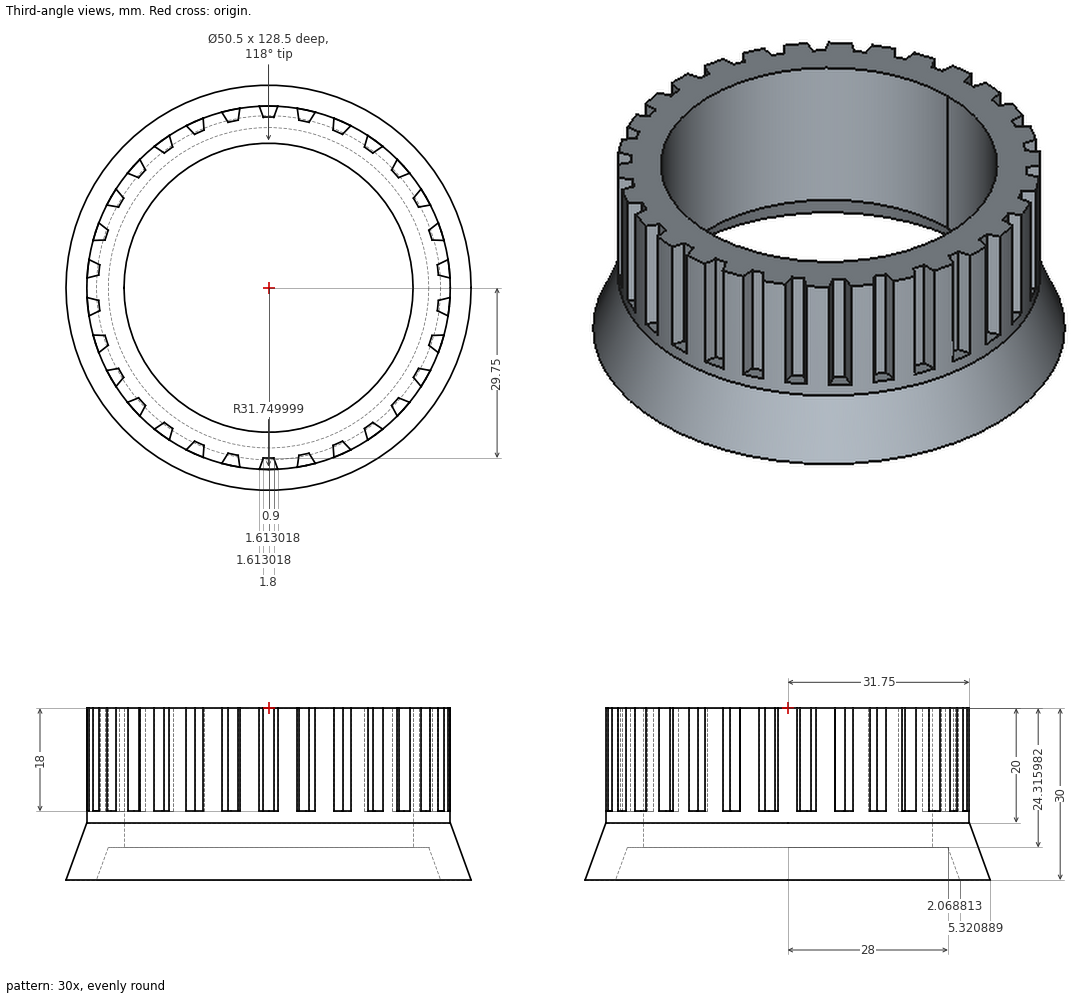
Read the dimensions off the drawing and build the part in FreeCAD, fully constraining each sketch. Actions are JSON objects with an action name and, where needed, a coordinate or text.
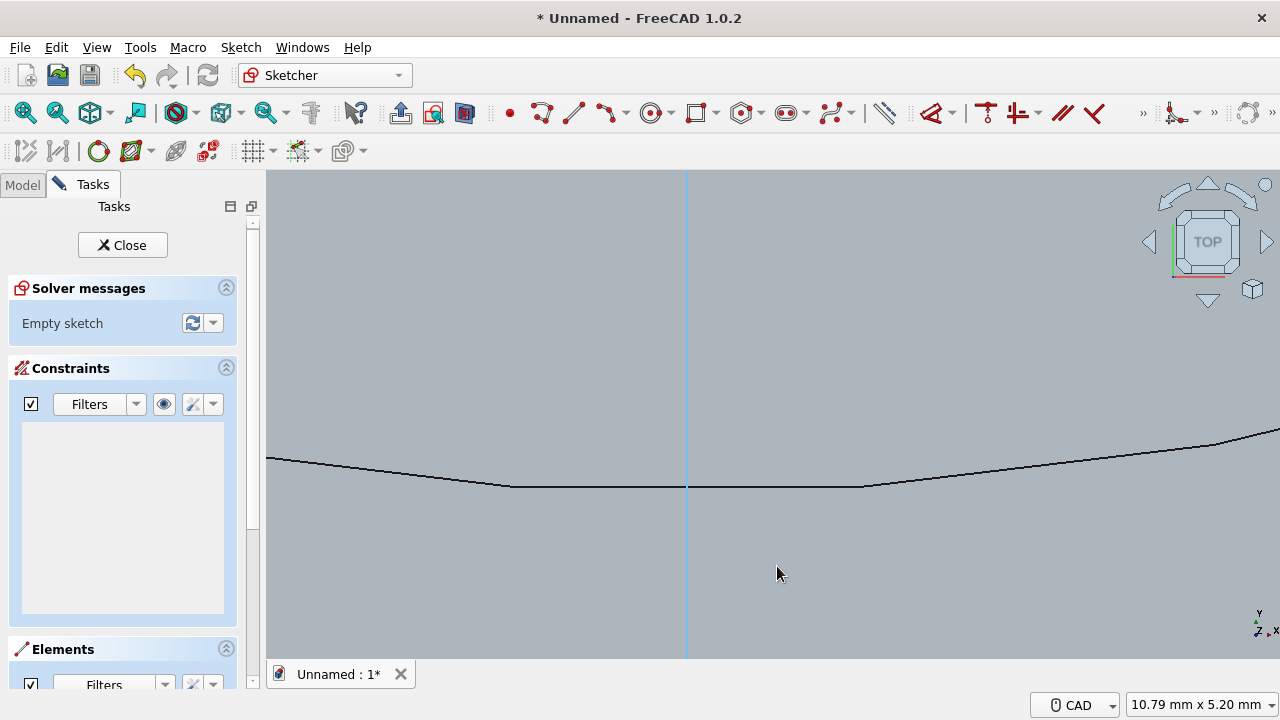
{"action": "scroll", "coordinate": [652, 364], "scroll_direction": "up", "scroll_amount": 2}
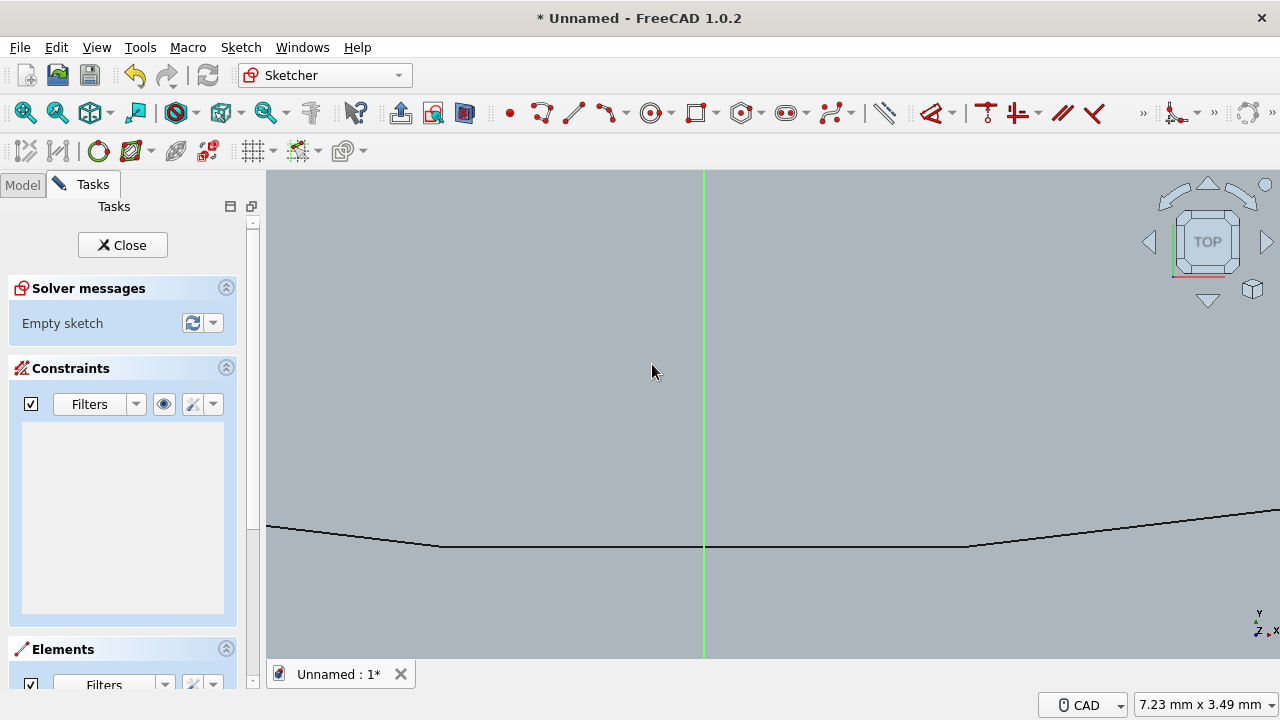
{"action": "left_click", "coordinate": [542, 114]}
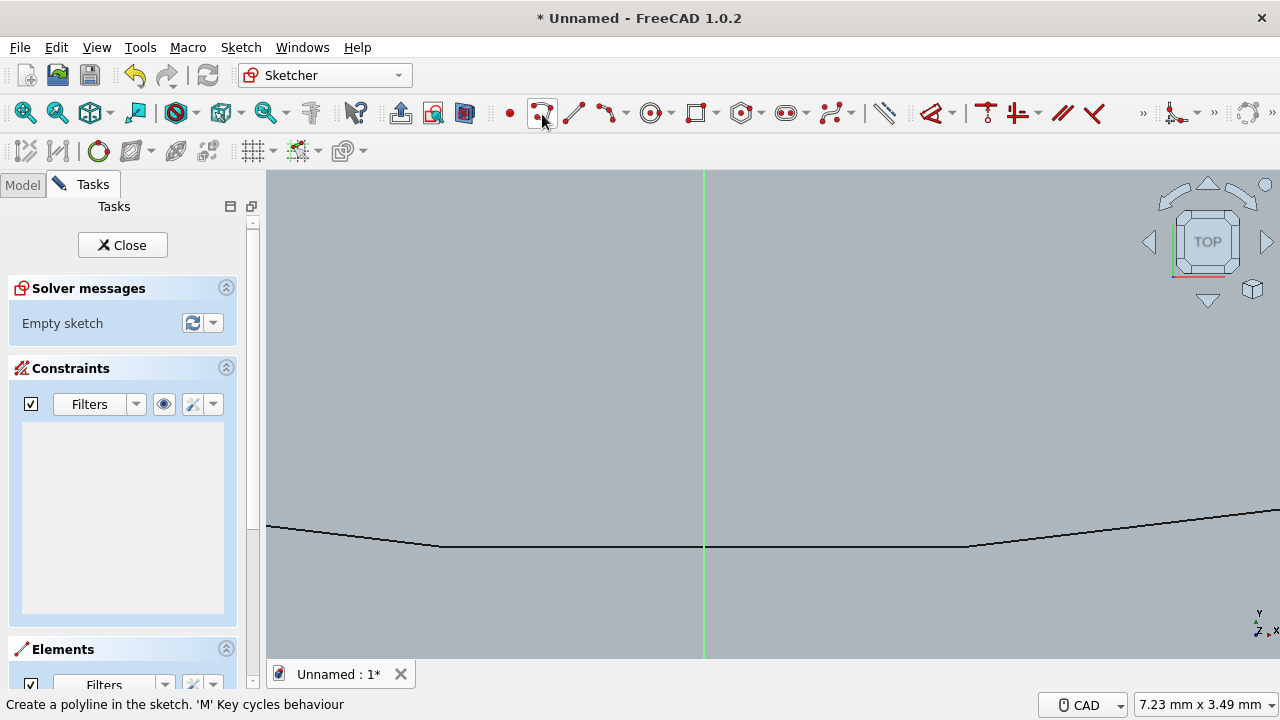
{"action": "left_click", "coordinate": [930, 549]}
{"action": "left_click", "coordinate": [830, 274]}
{"action": "left_click", "coordinate": [578, 274]}
{"action": "left_click", "coordinate": [478, 549]}
{"action": "right_click", "coordinate": [478, 549]}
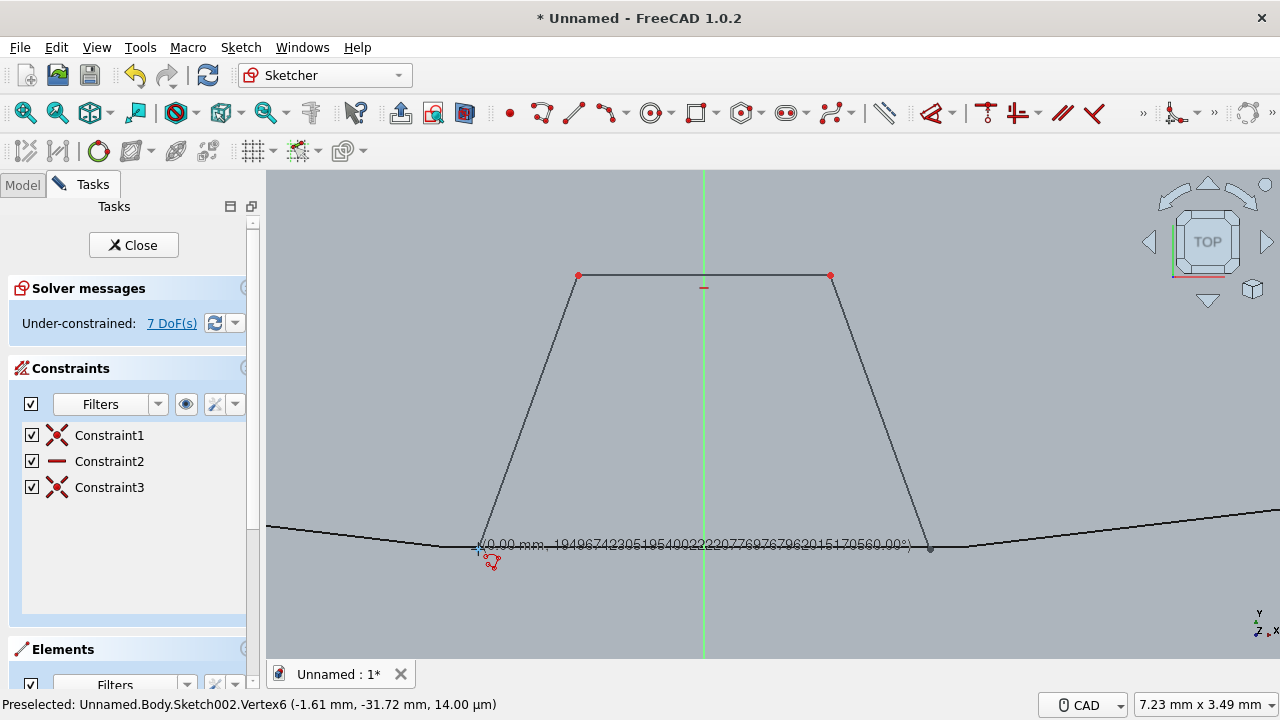
{"action": "left_click", "coordinate": [606, 114]}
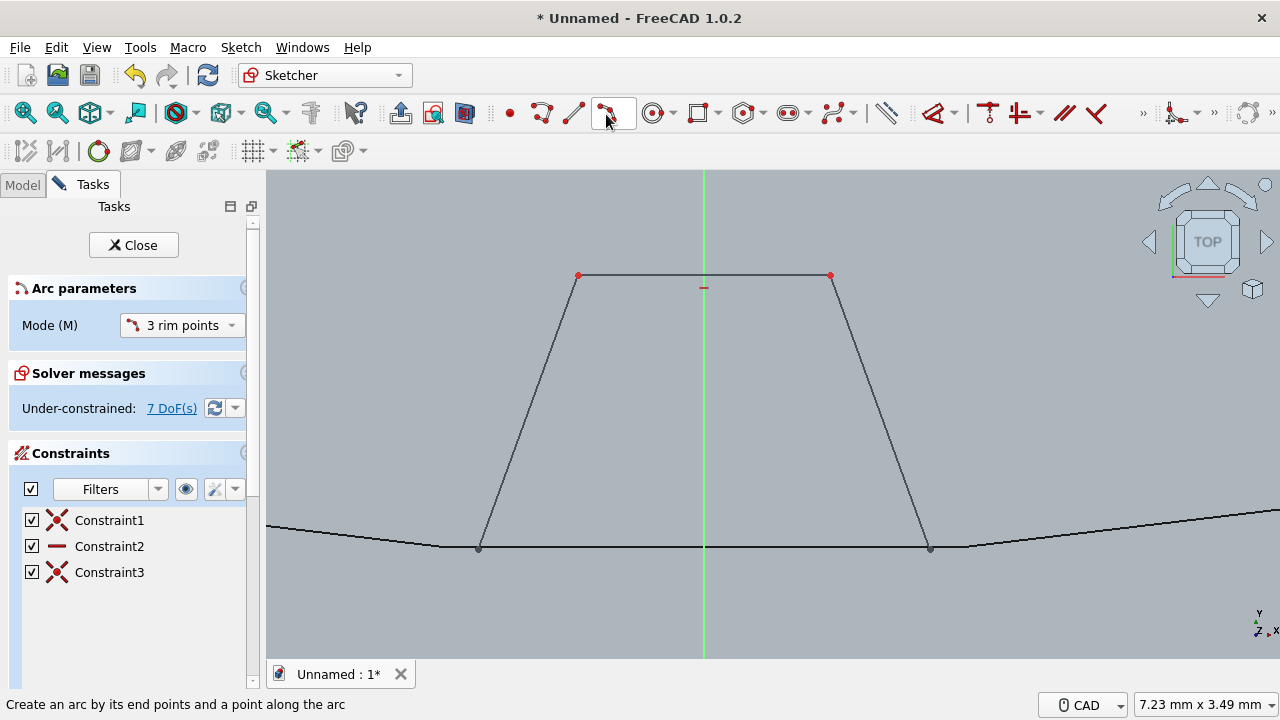
{"action": "left_click", "coordinate": [478, 550]}
{"action": "left_click", "coordinate": [930, 550]}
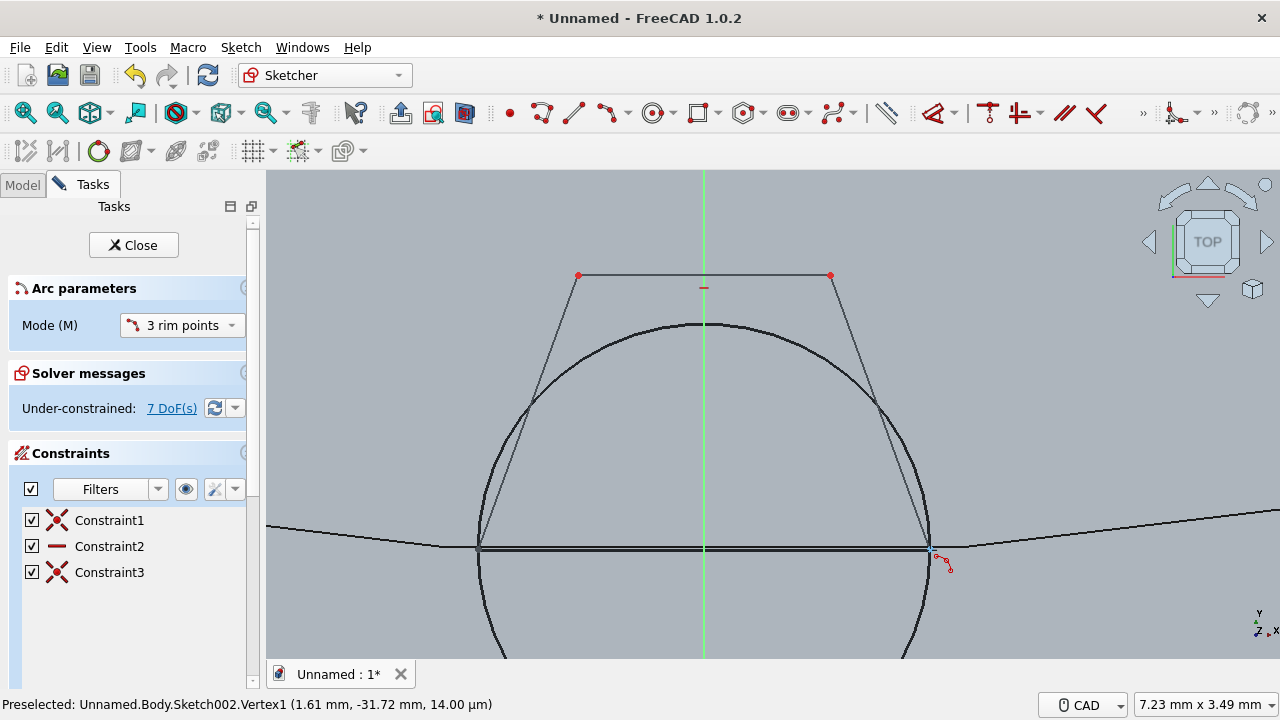
{"action": "scroll", "coordinate": [659, 554], "scroll_direction": "up", "scroll_amount": 6}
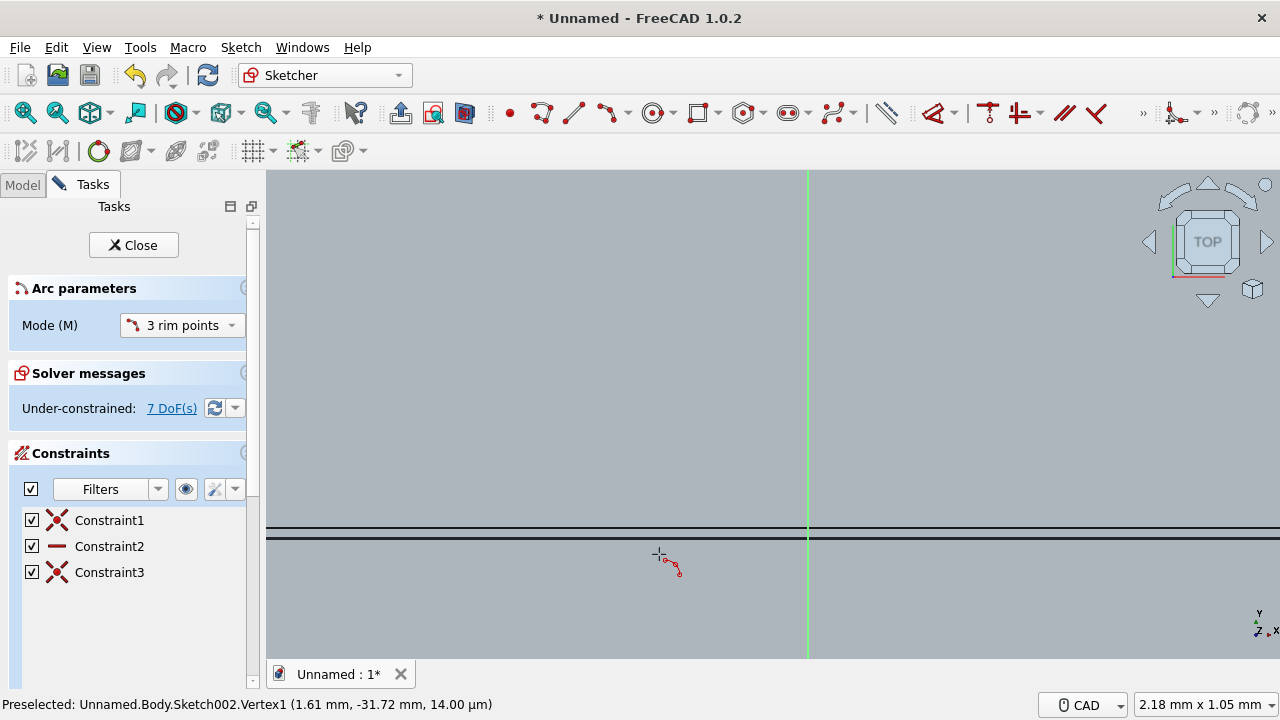
{"action": "left_click", "coordinate": [657, 553]}
{"action": "key", "text": "Escape"}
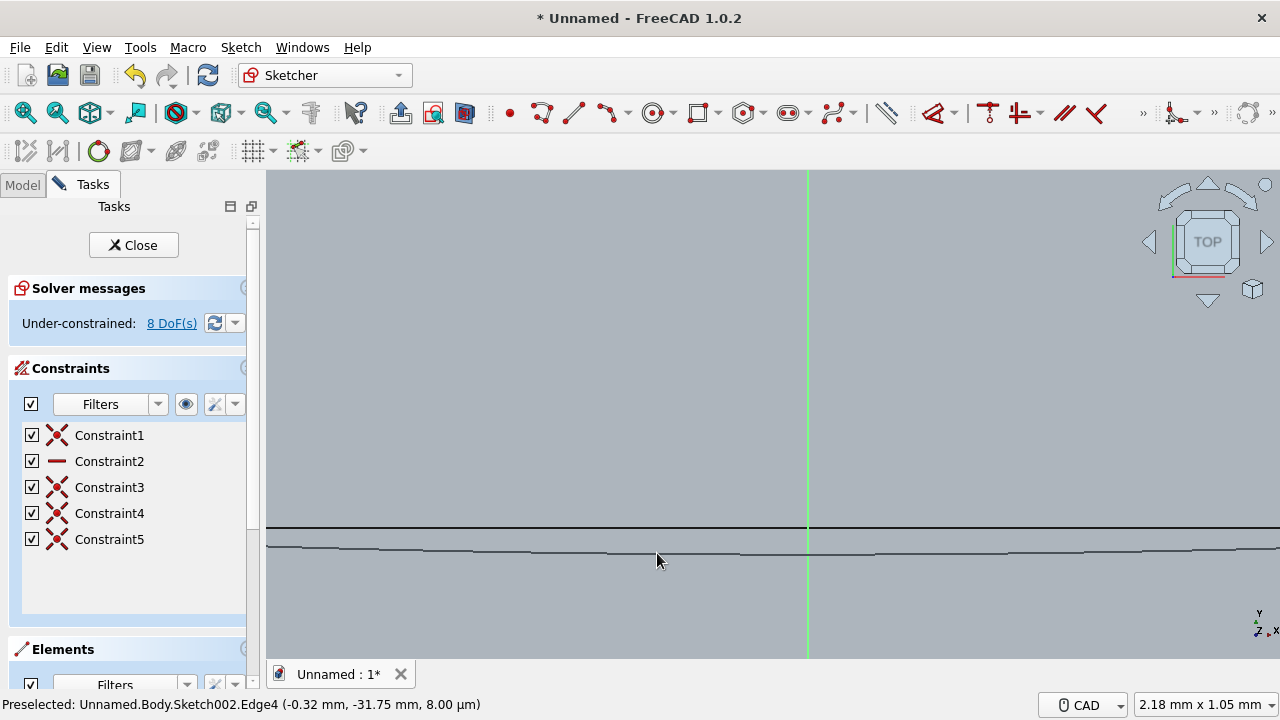
{"action": "scroll", "coordinate": [660, 555], "scroll_direction": "down", "scroll_amount": 6}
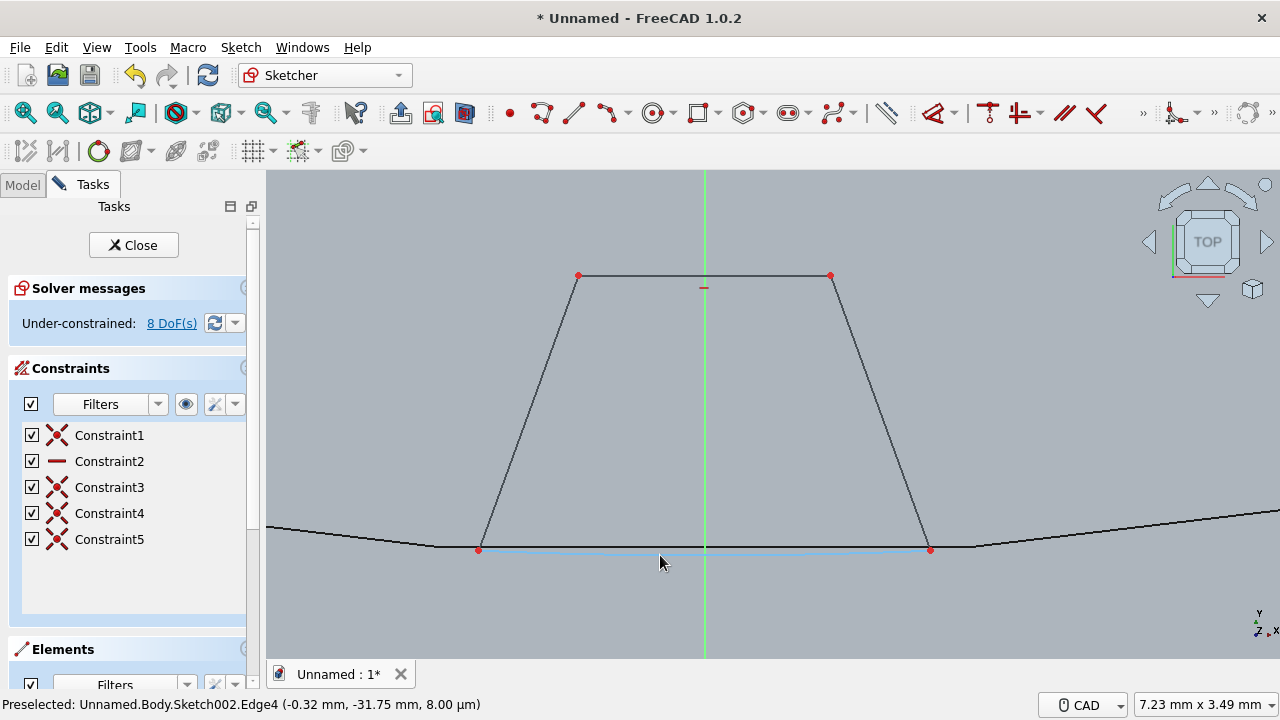
{"action": "scroll", "coordinate": [704, 565], "scroll_direction": "down", "scroll_amount": 14}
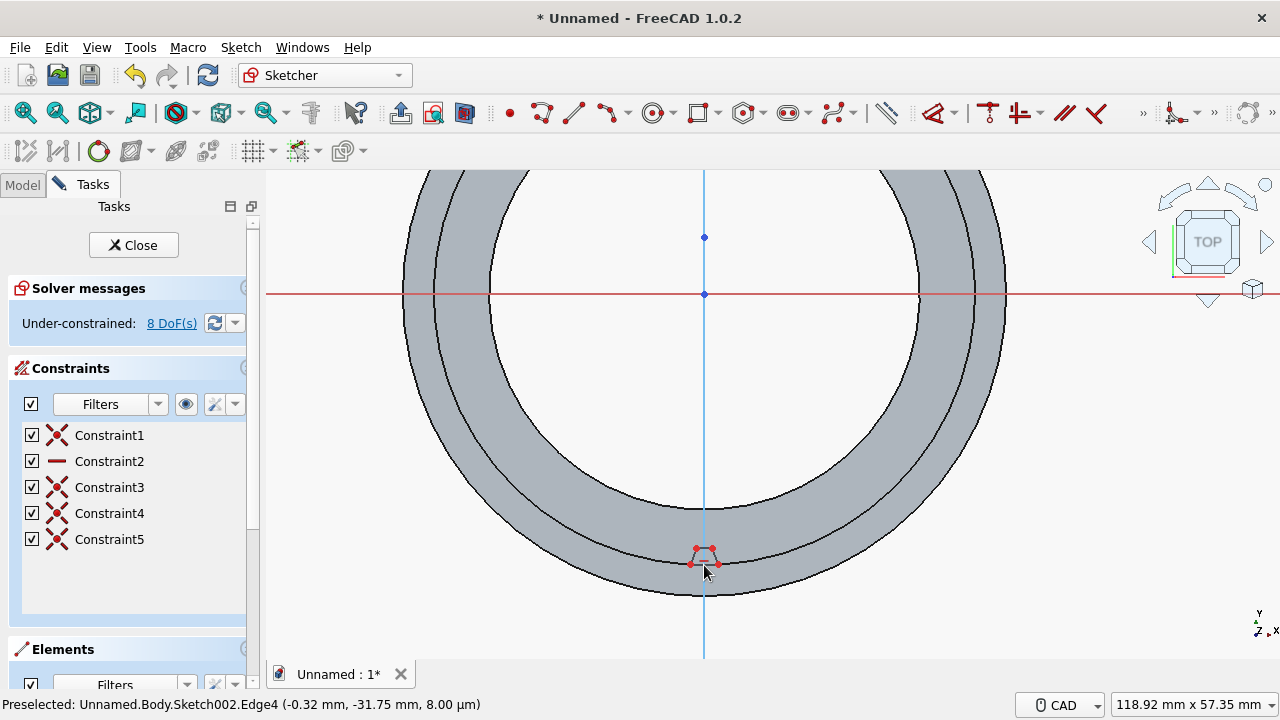
{"action": "left_click_drag", "start_coordinate": [694, 228], "coordinate": [714, 304]}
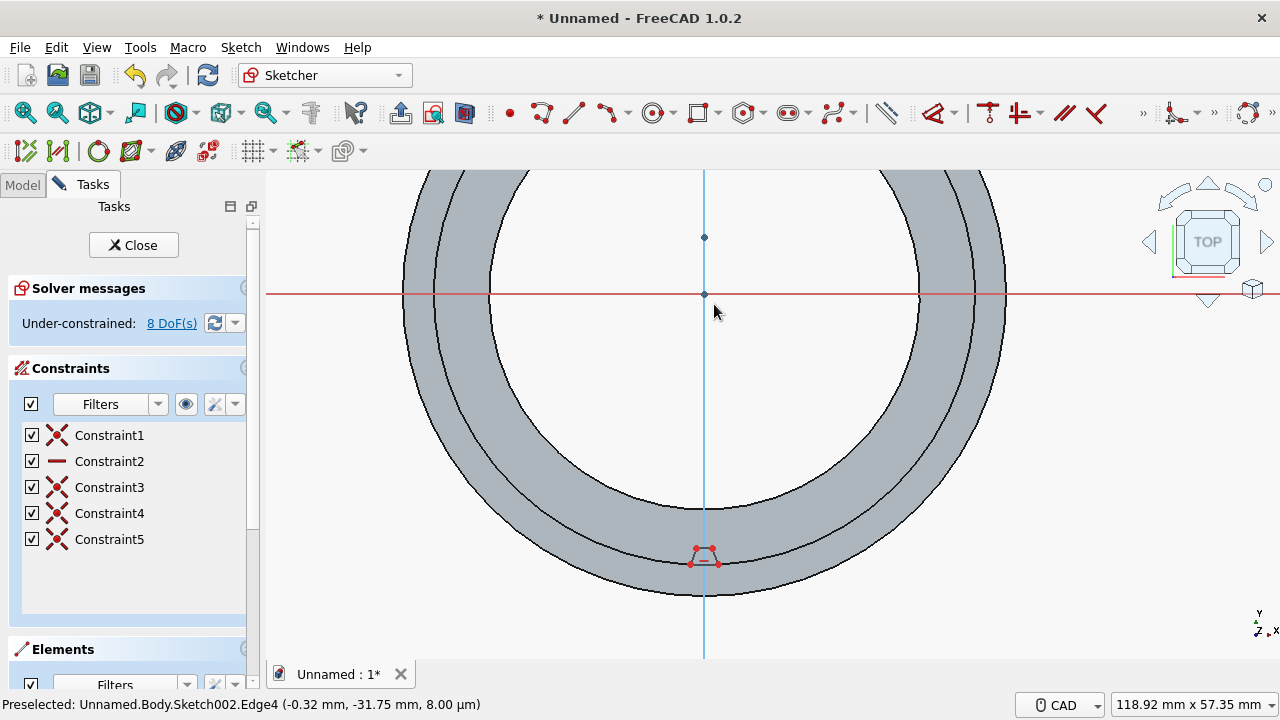
{"action": "key", "text": "c"}